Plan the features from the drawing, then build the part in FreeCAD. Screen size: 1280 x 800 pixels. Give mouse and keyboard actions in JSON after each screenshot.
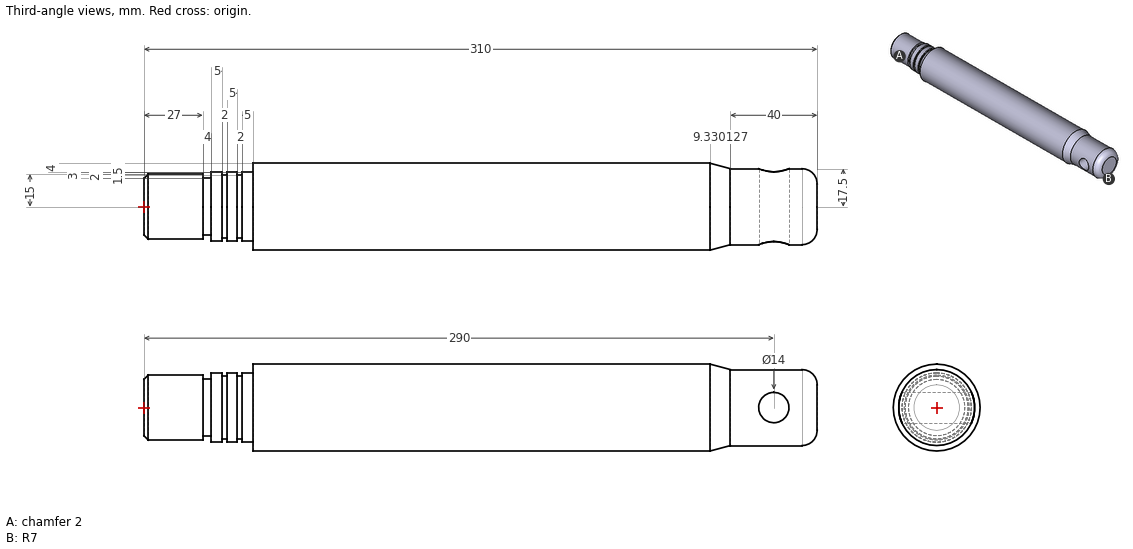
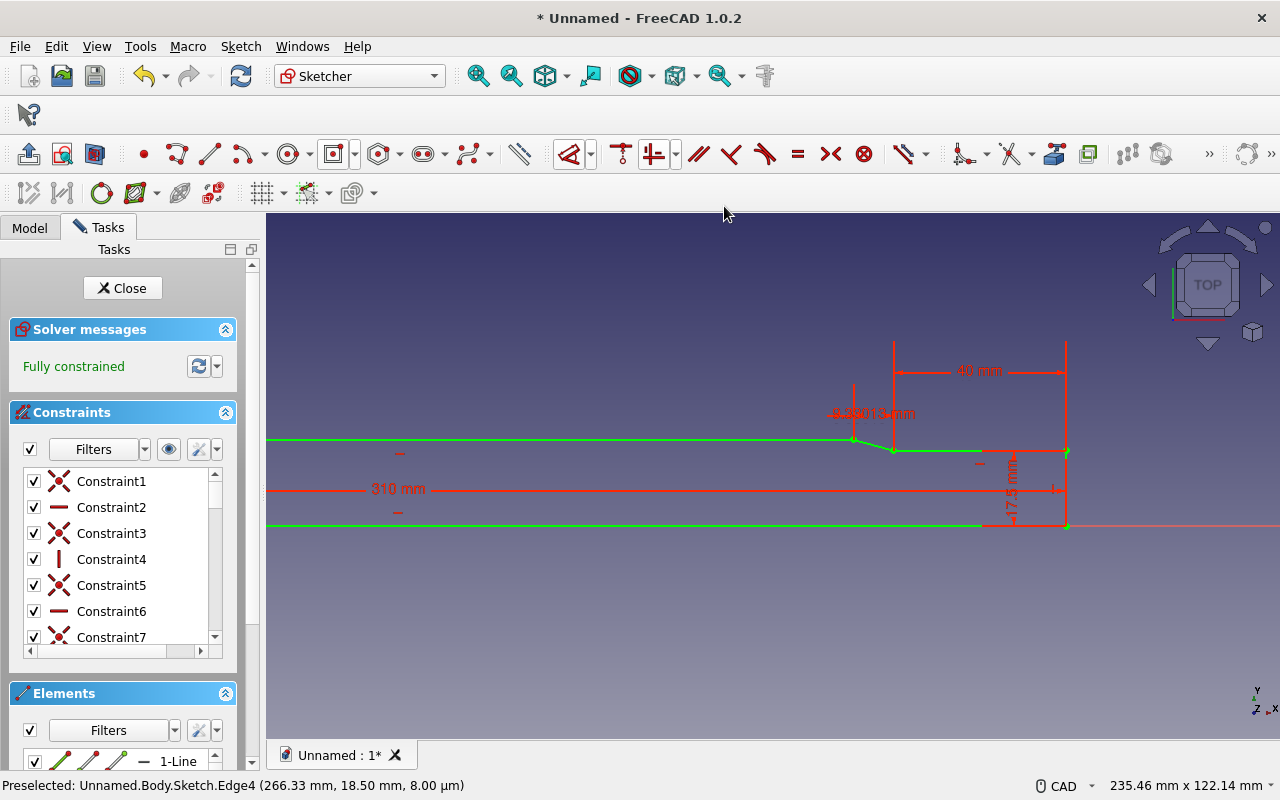
{"action": "left_click", "coordinate": [123, 288]}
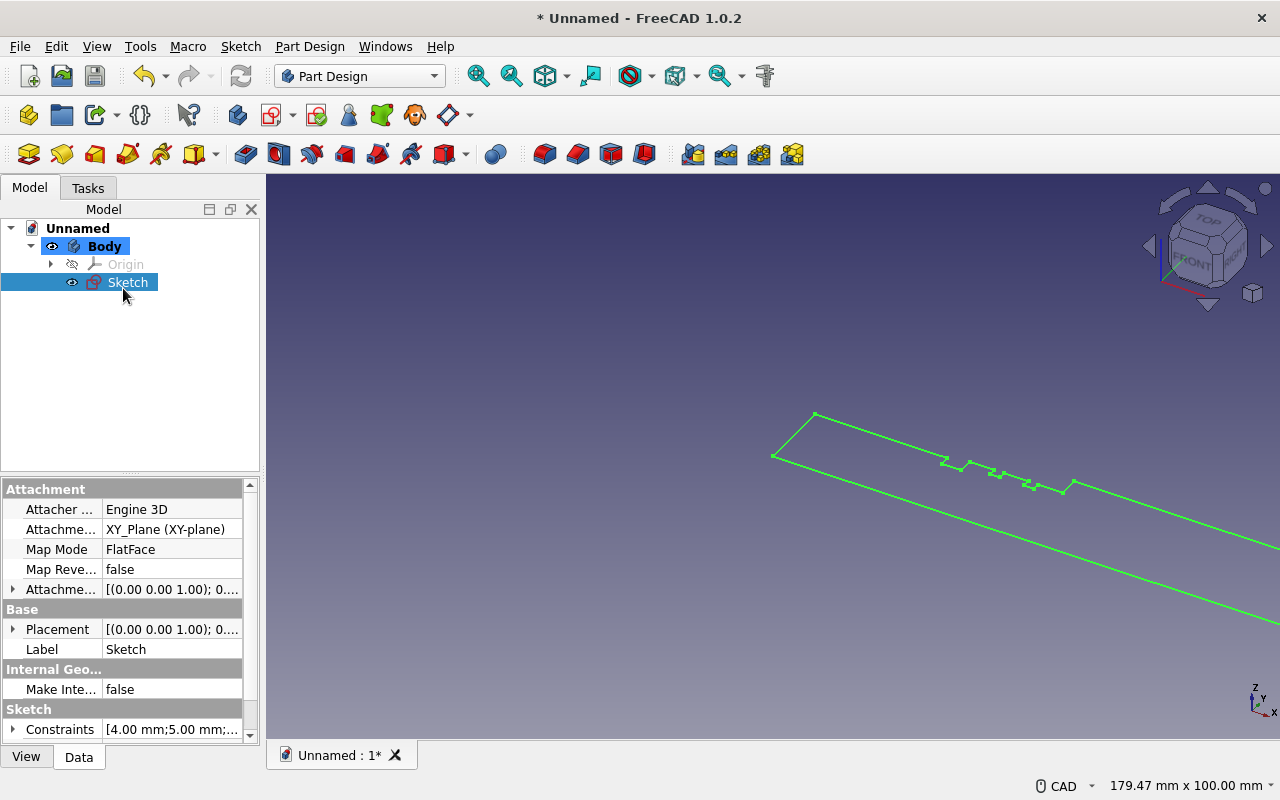
{"action": "left_click", "coordinate": [62, 154]}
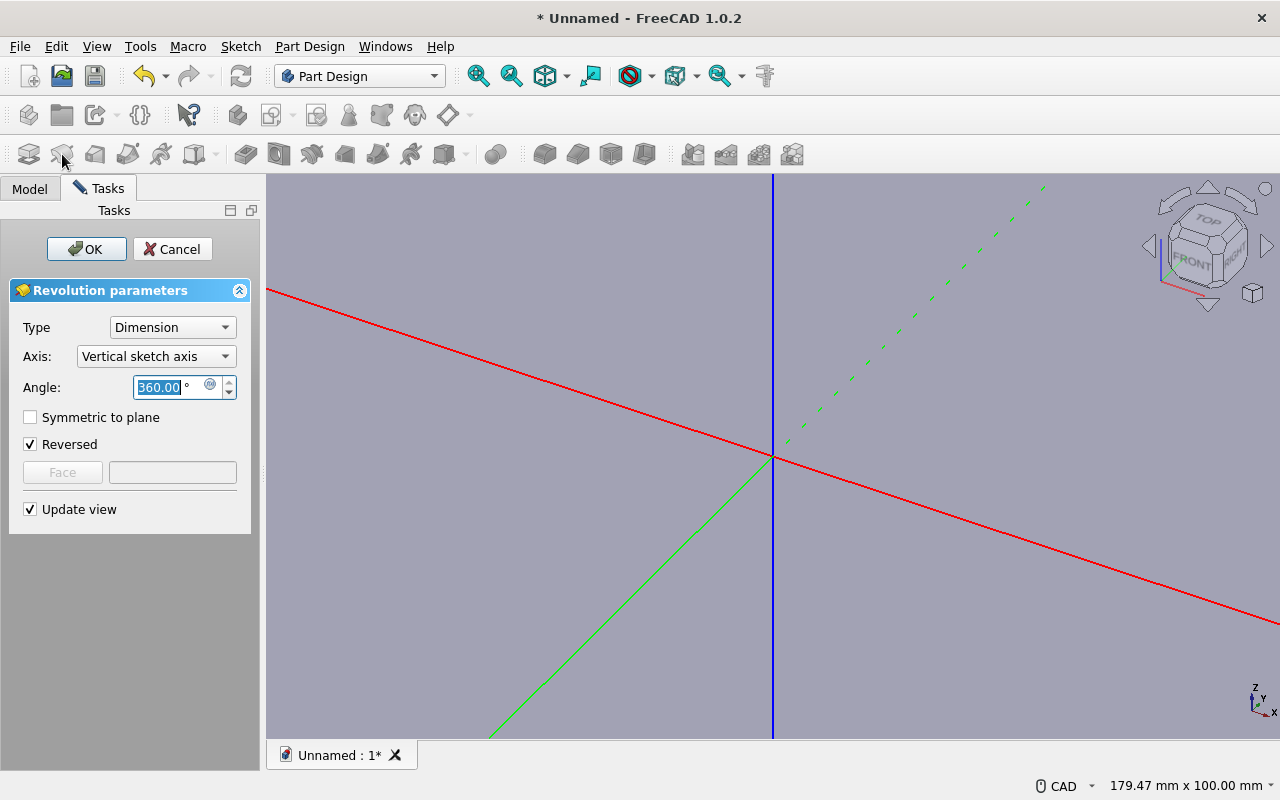
{"action": "left_click", "coordinate": [157, 356]}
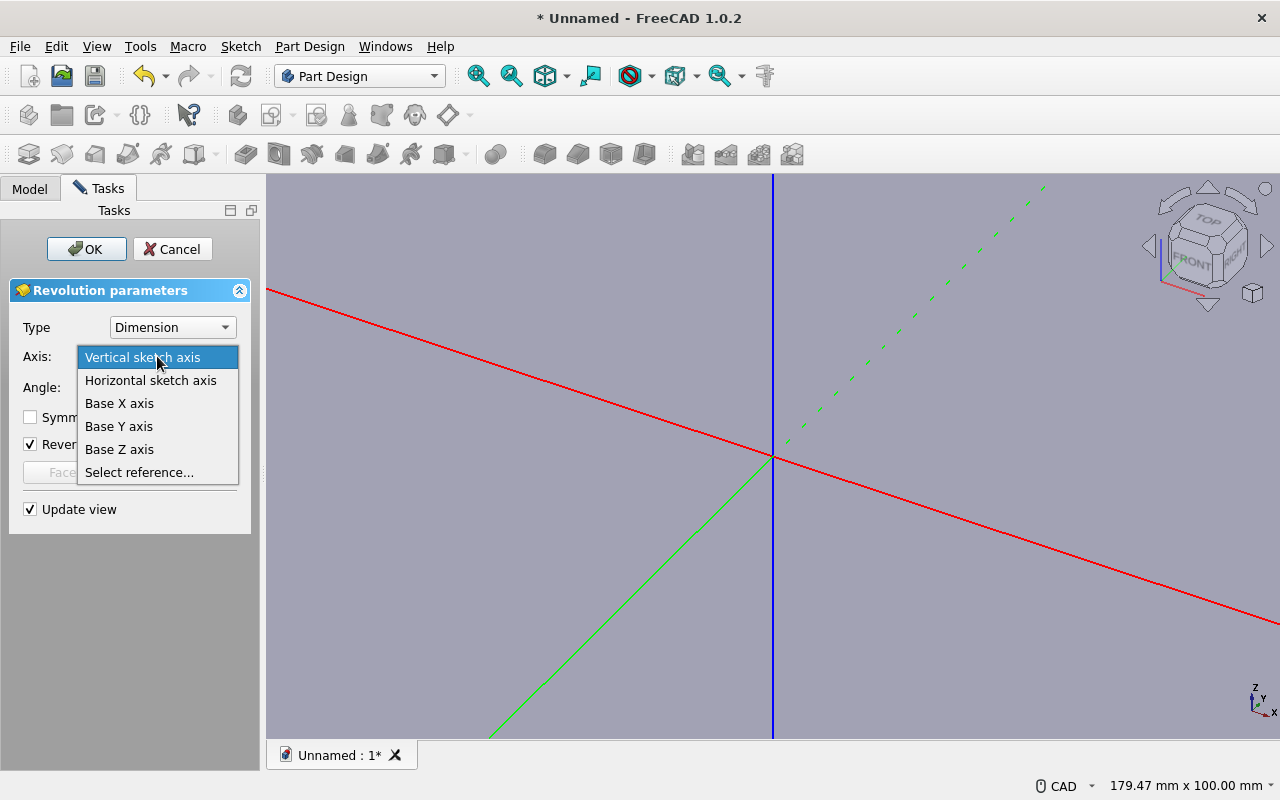
{"action": "left_click", "coordinate": [156, 380]}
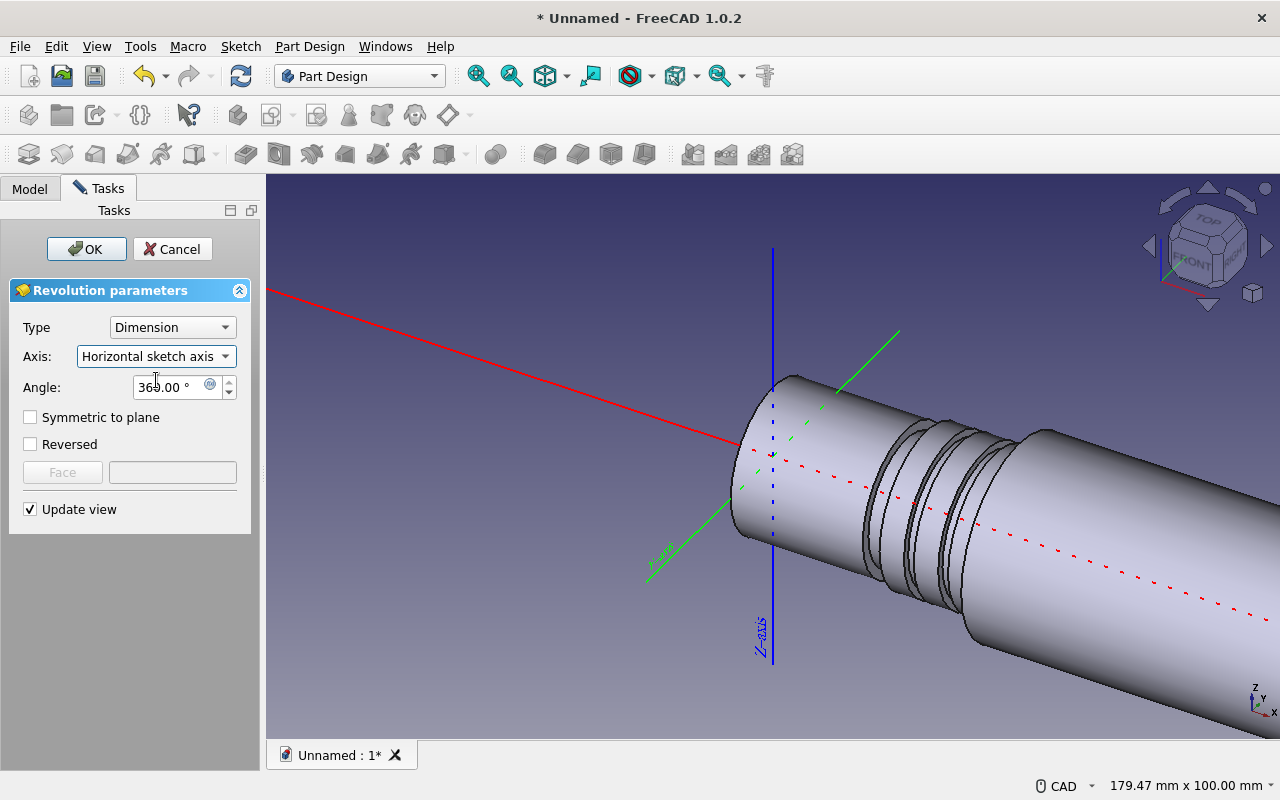
{"action": "left_click", "coordinate": [87, 249]}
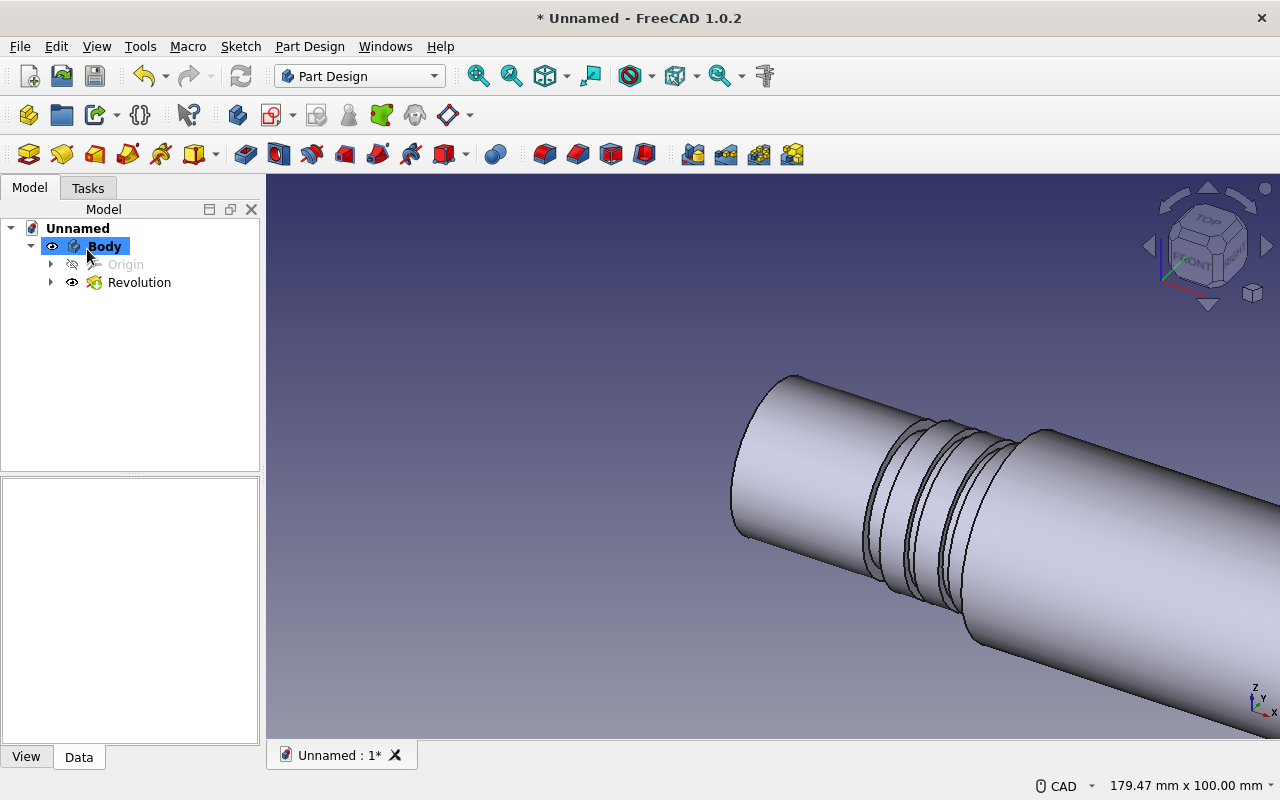
{"action": "left_click", "coordinate": [479, 76]}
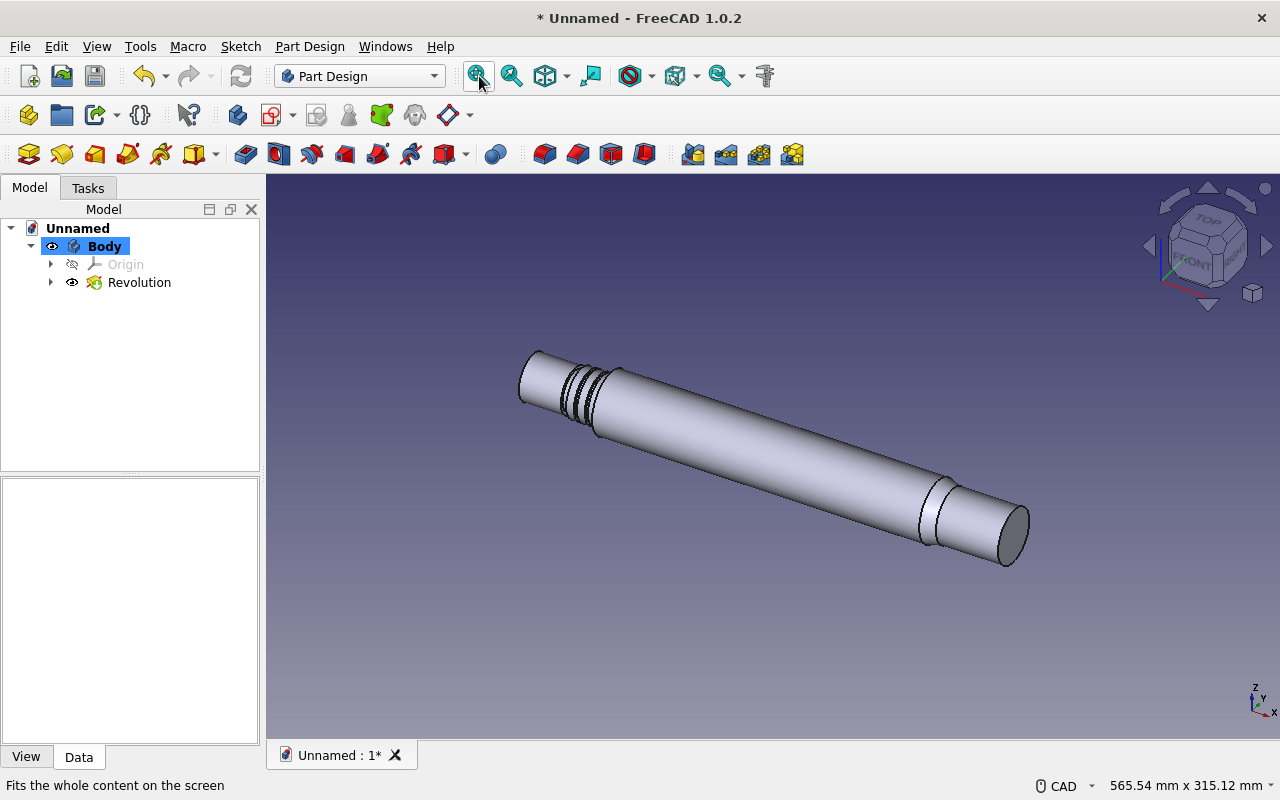
{"action": "left_click", "coordinate": [270, 116]}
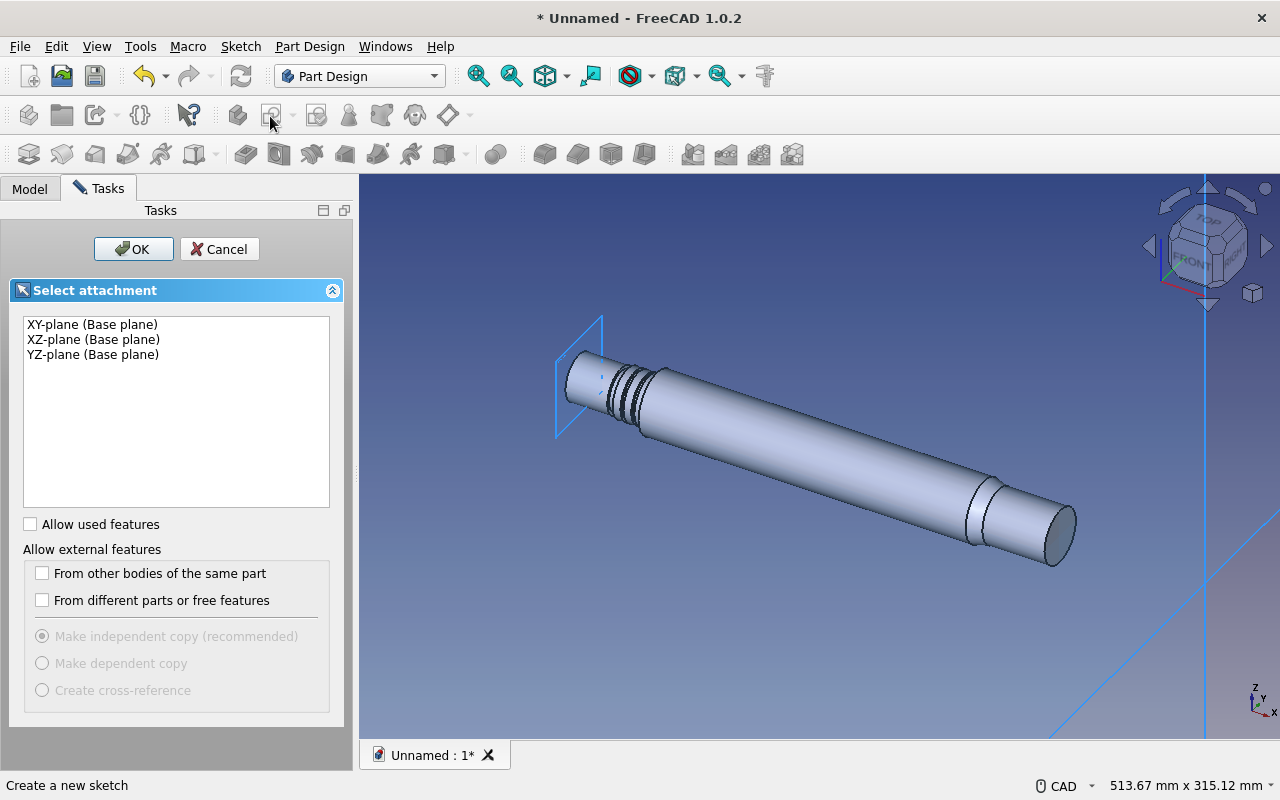
{"action": "left_click", "coordinate": [84, 340]}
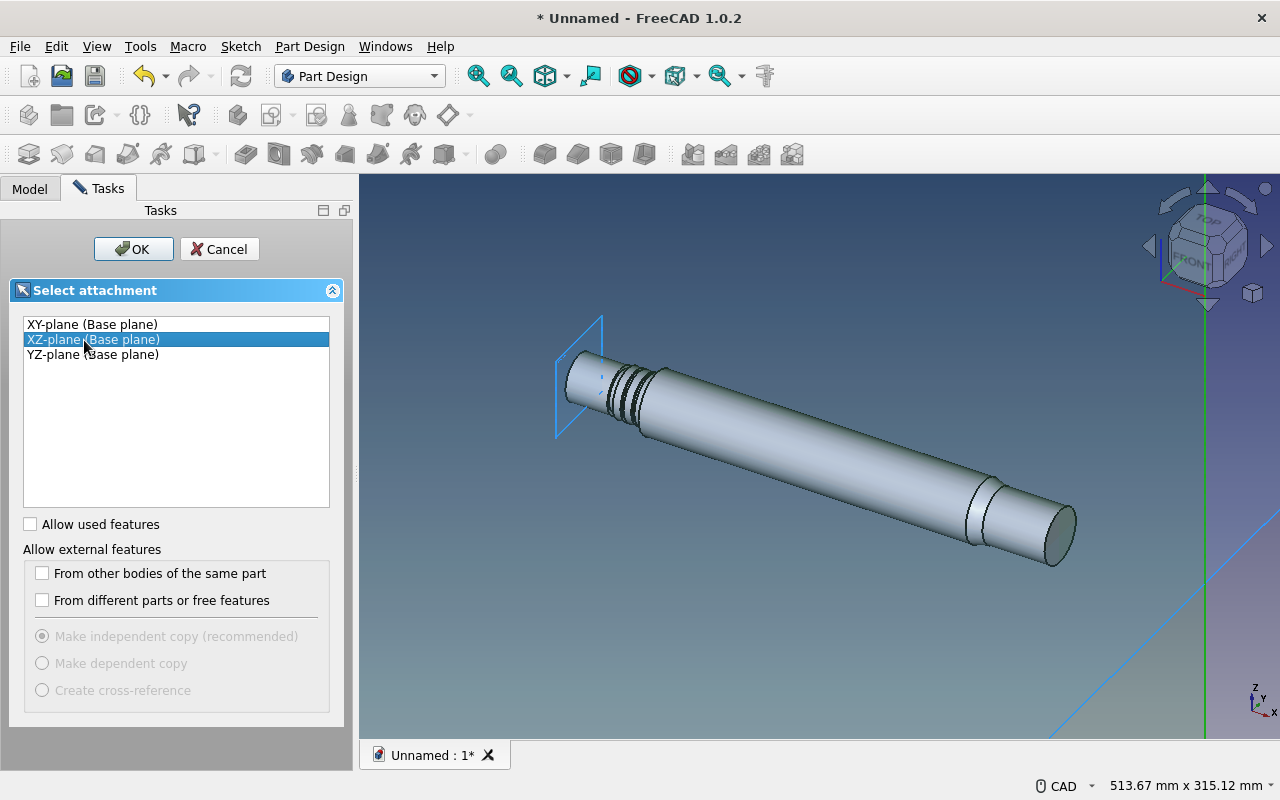
{"action": "left_click", "coordinate": [134, 249]}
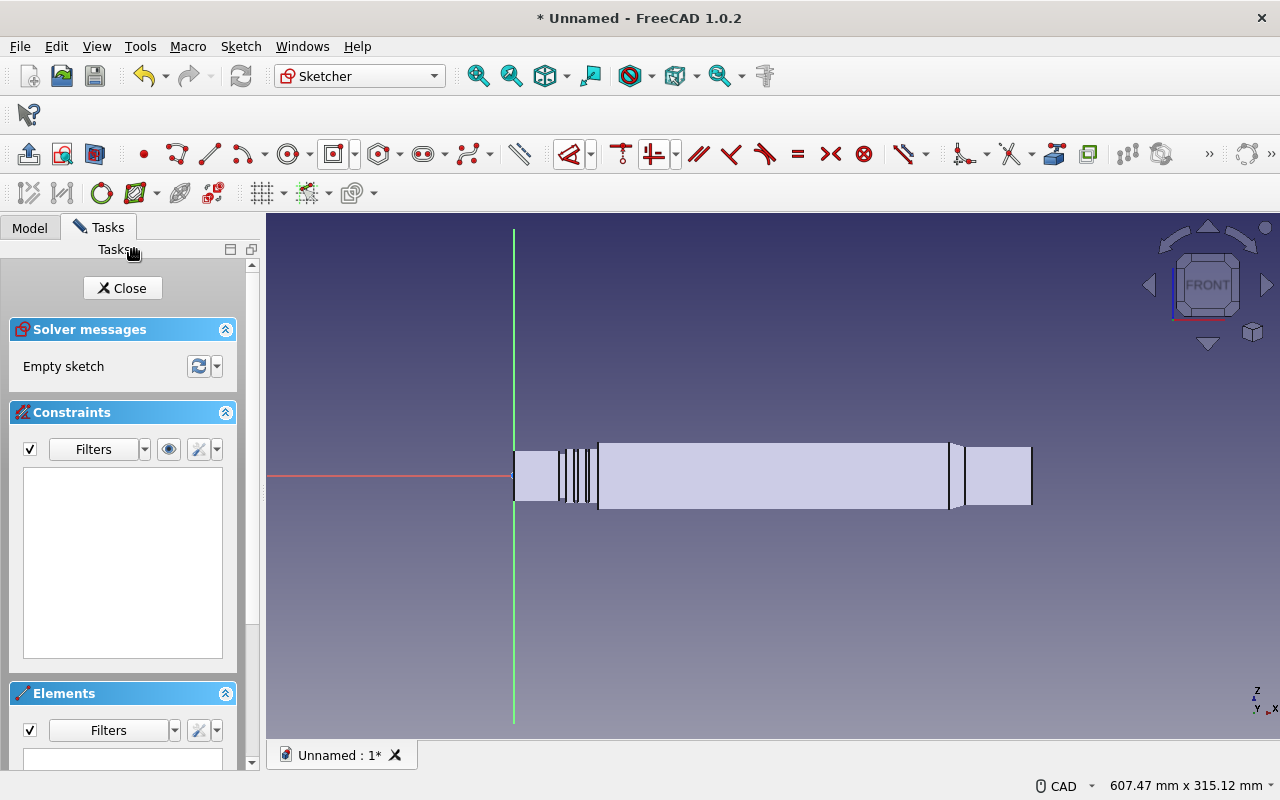
{"action": "left_click", "coordinate": [95, 154]}